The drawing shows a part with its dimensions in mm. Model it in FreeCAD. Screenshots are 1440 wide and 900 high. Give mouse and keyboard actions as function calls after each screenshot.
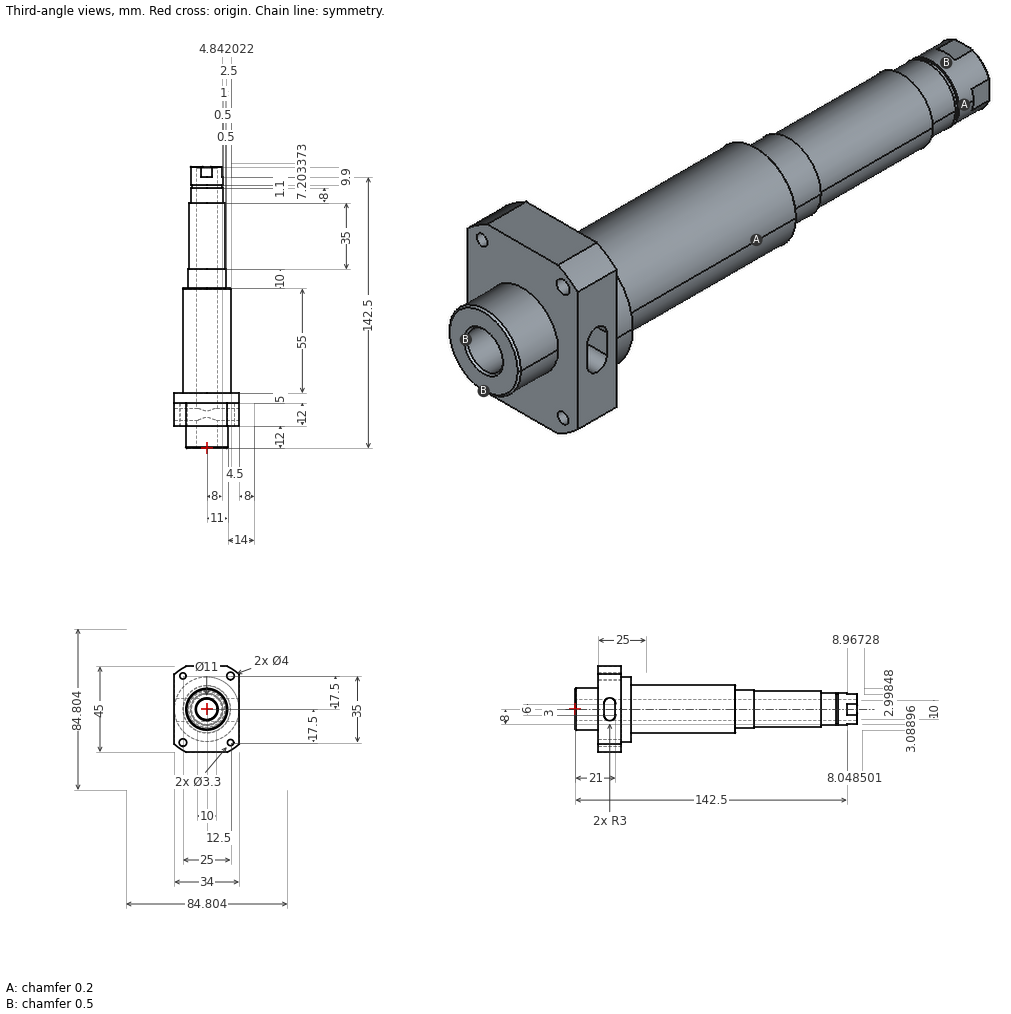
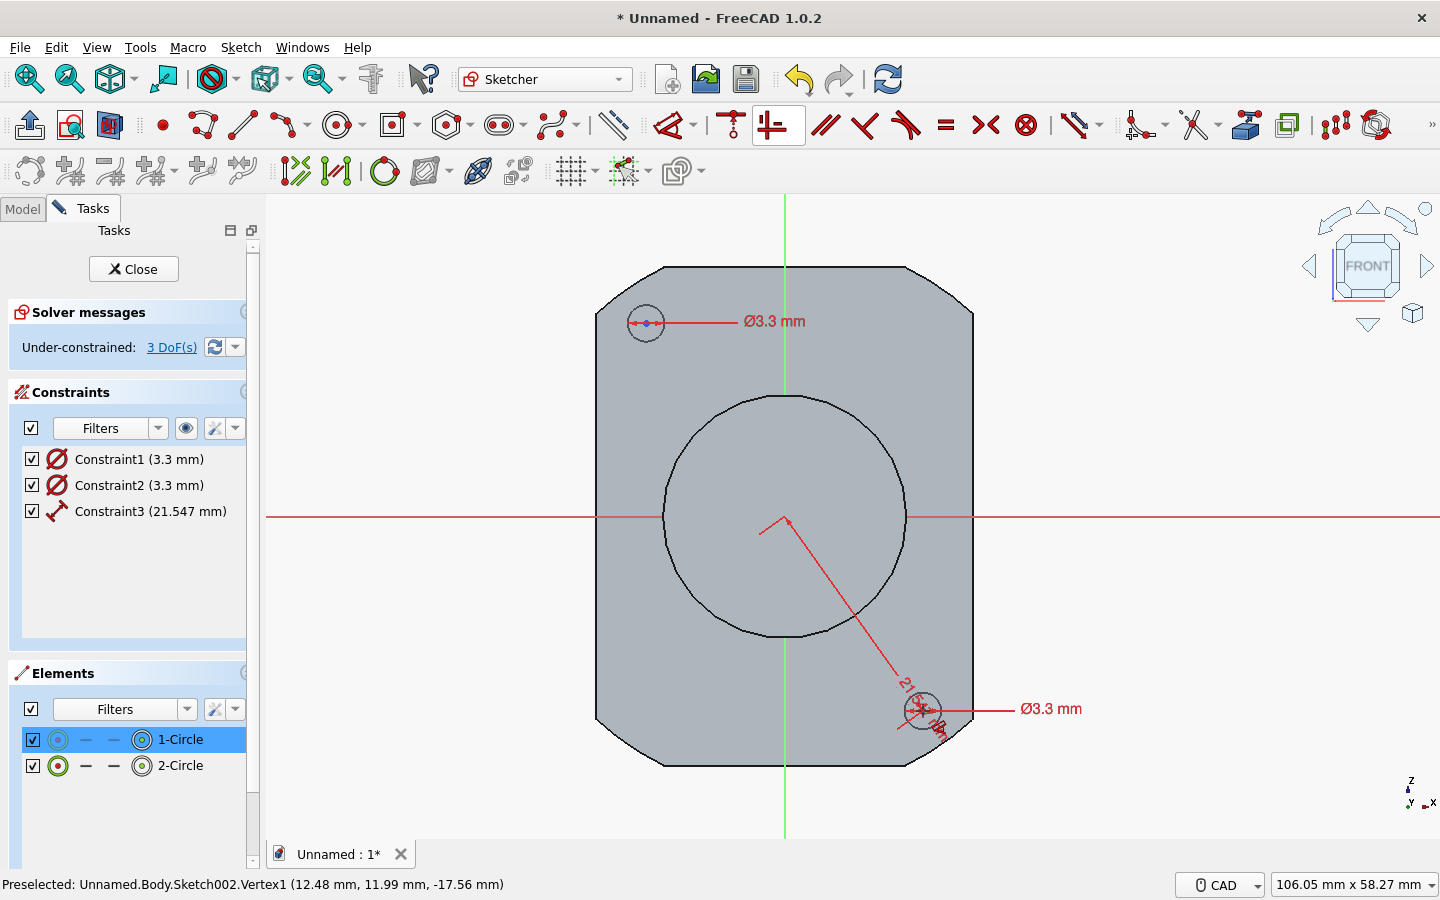
click(646, 323)
click(721, 745)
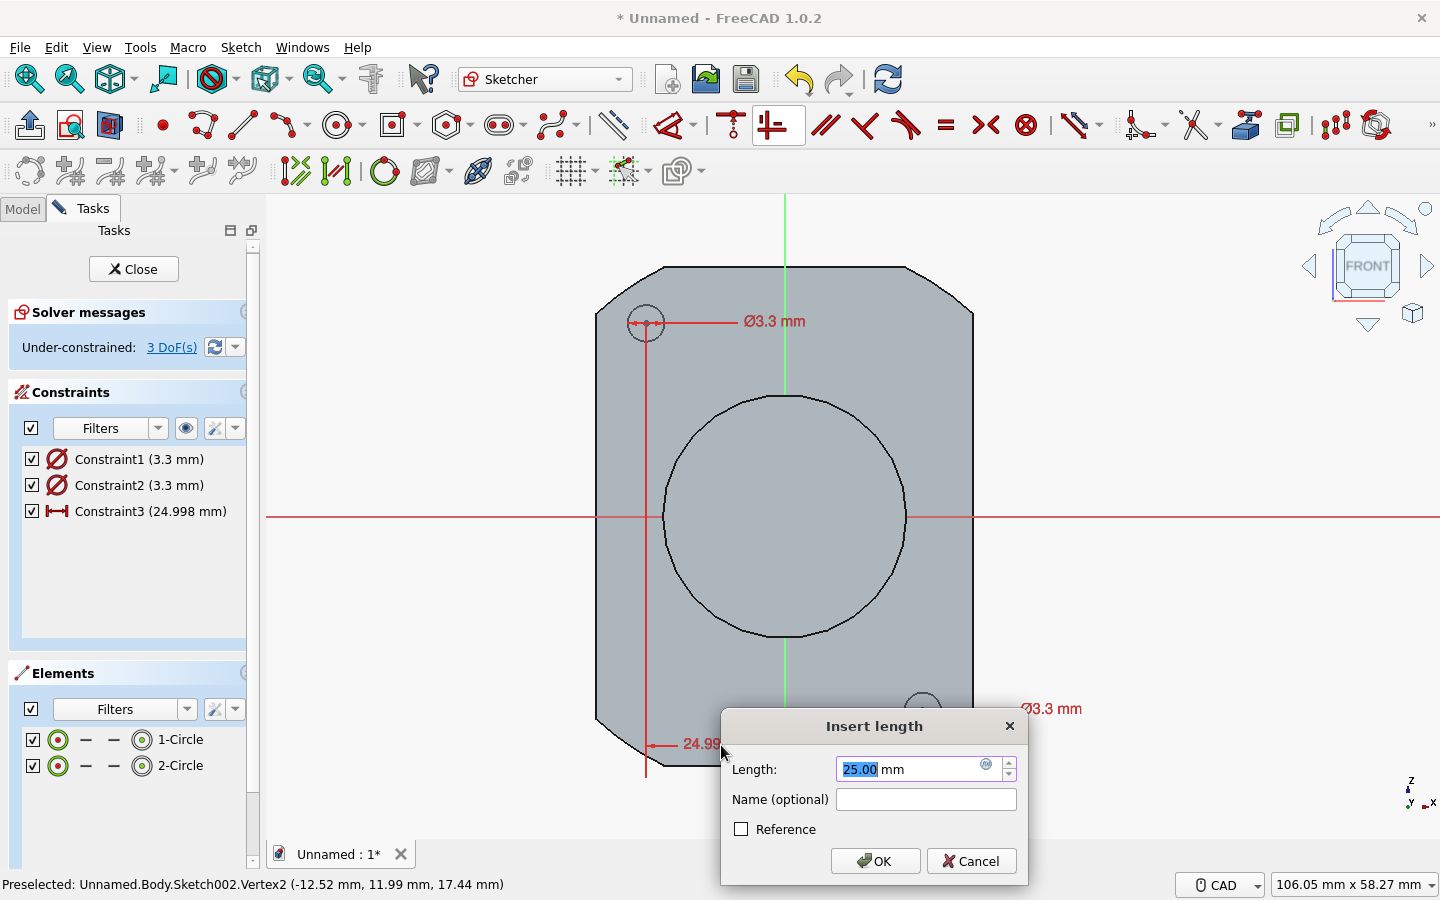
text(25)
key(Return)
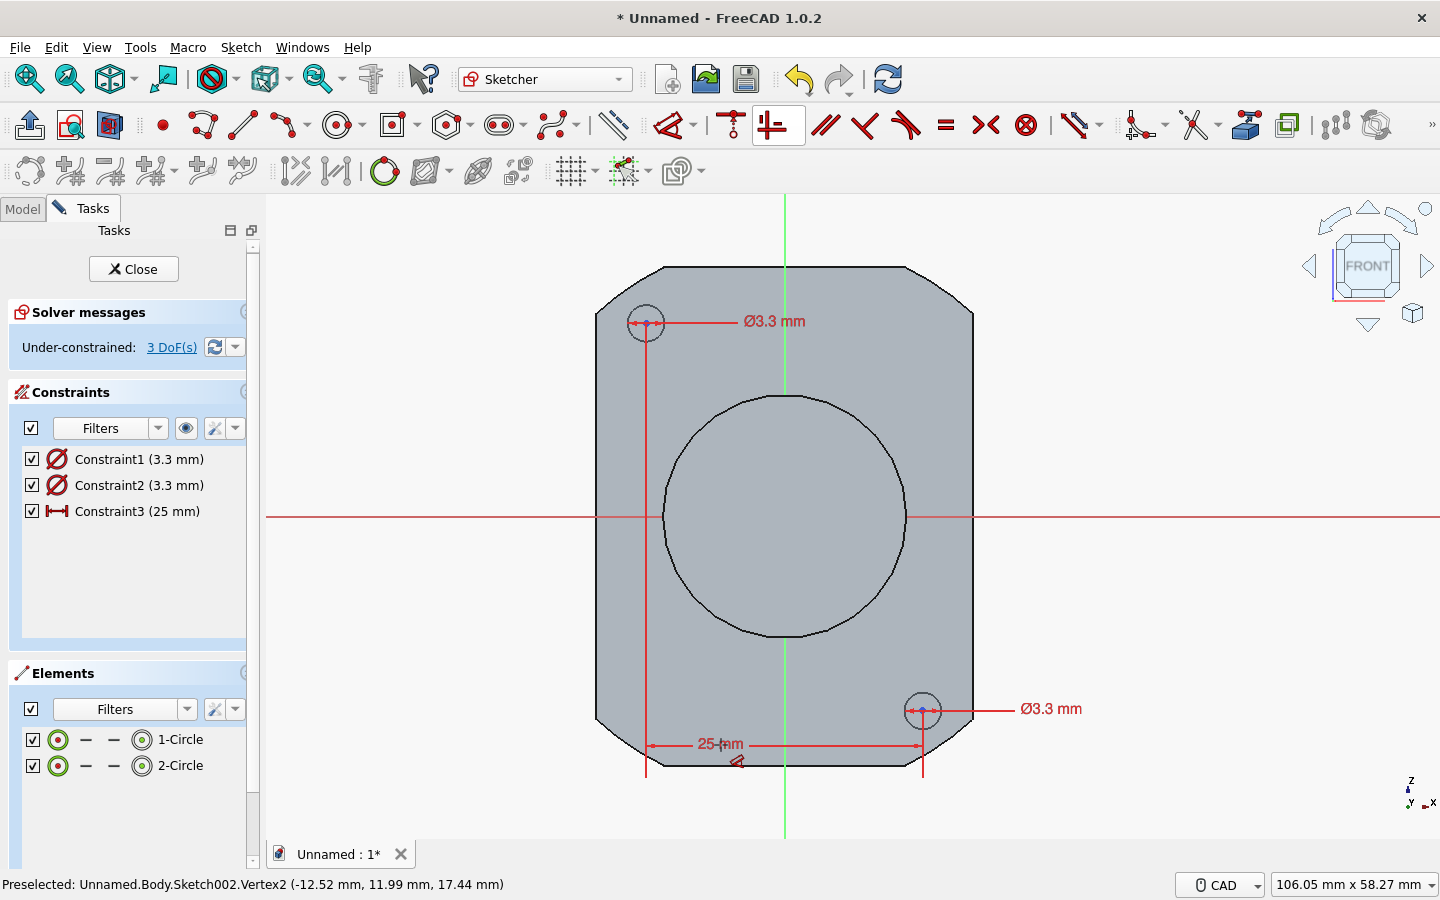
click(923, 711)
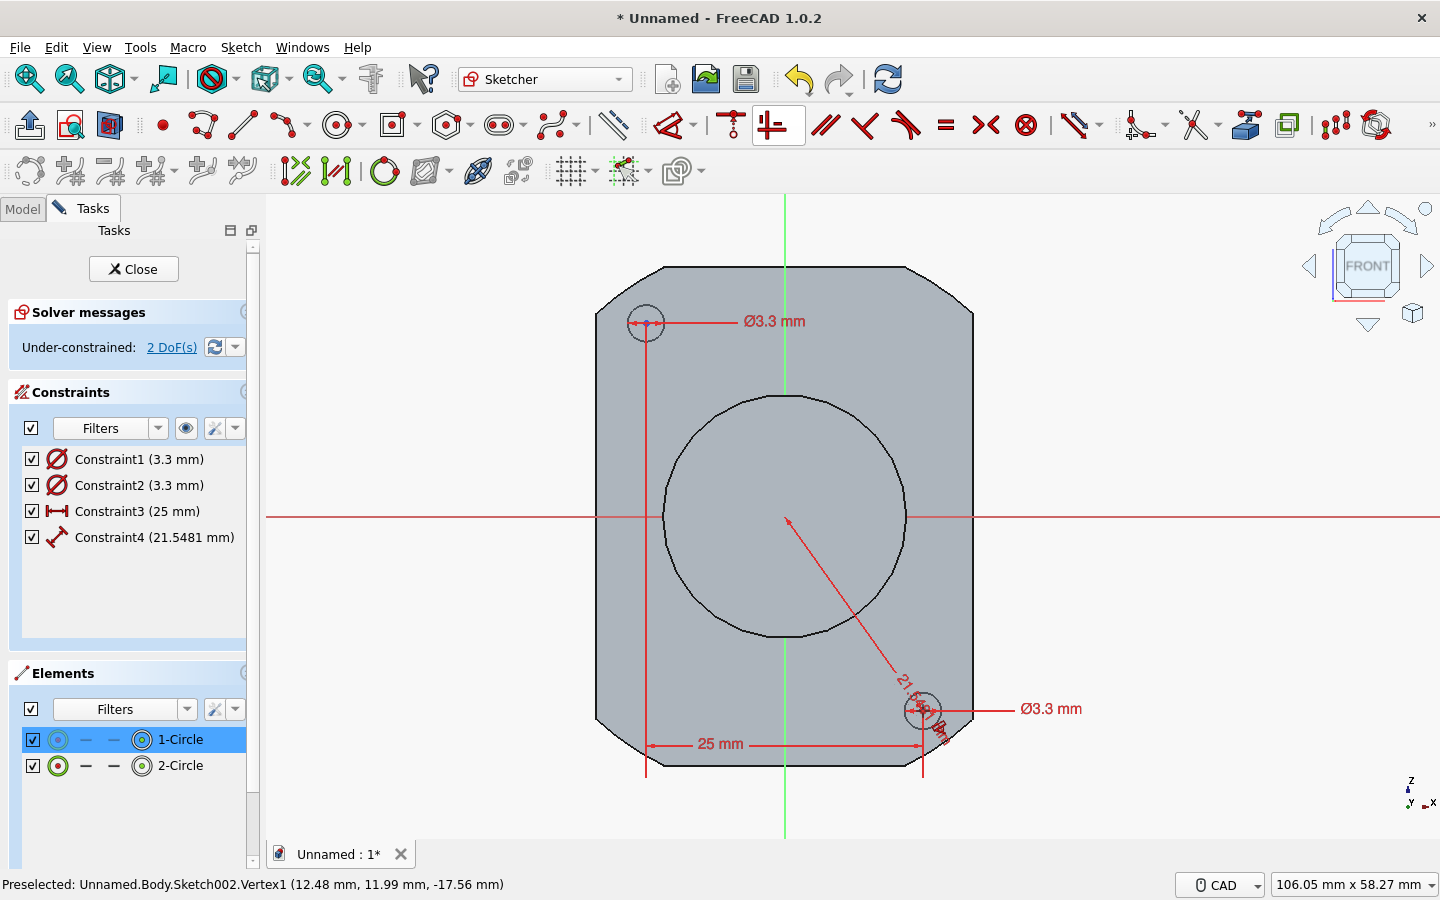
click(646, 323)
click(612, 428)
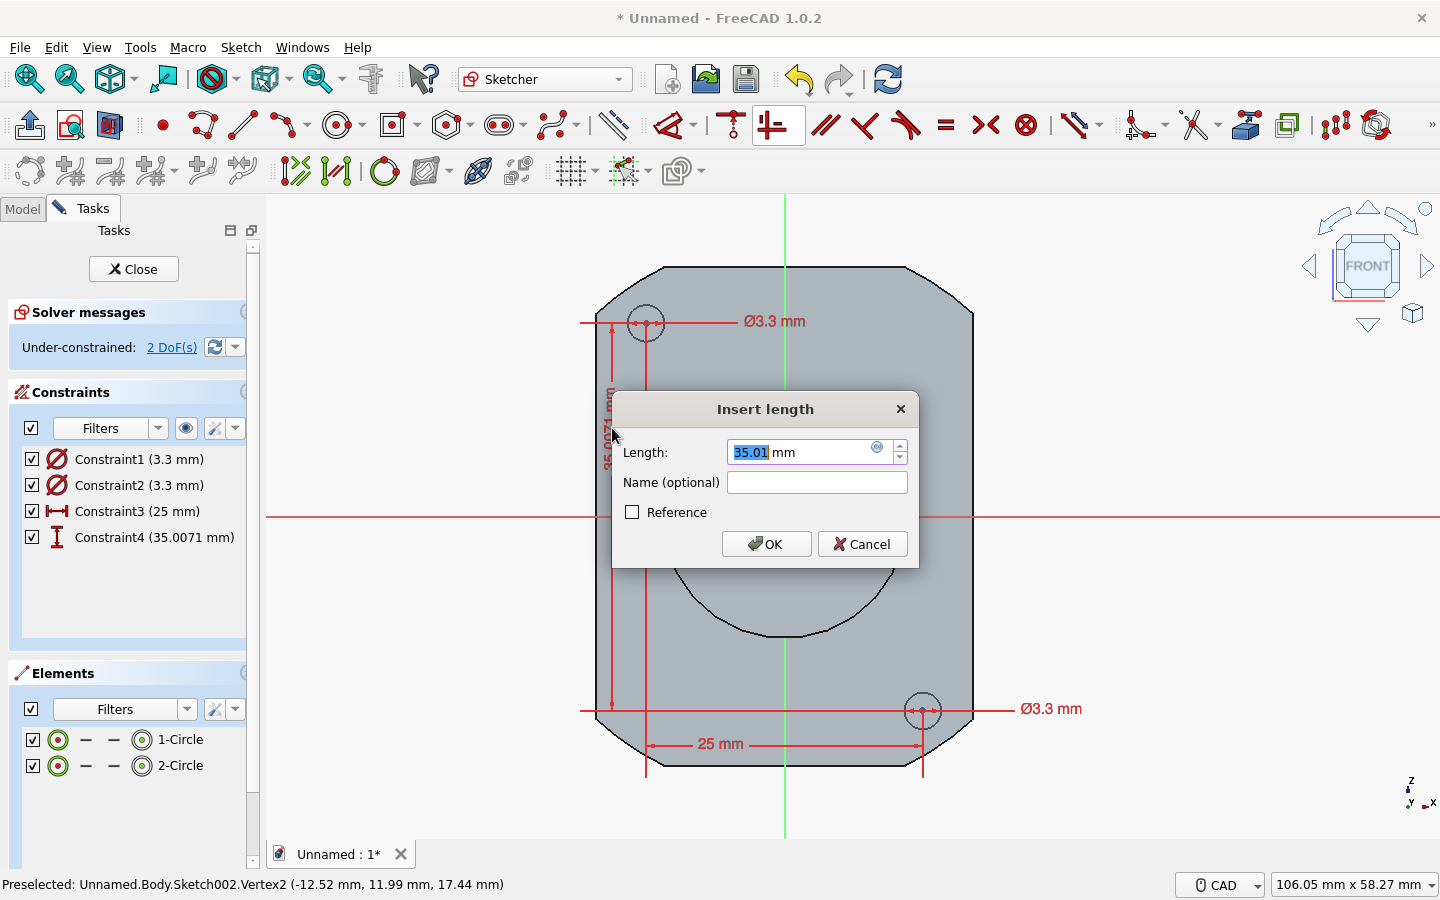
text(35)
key(Return)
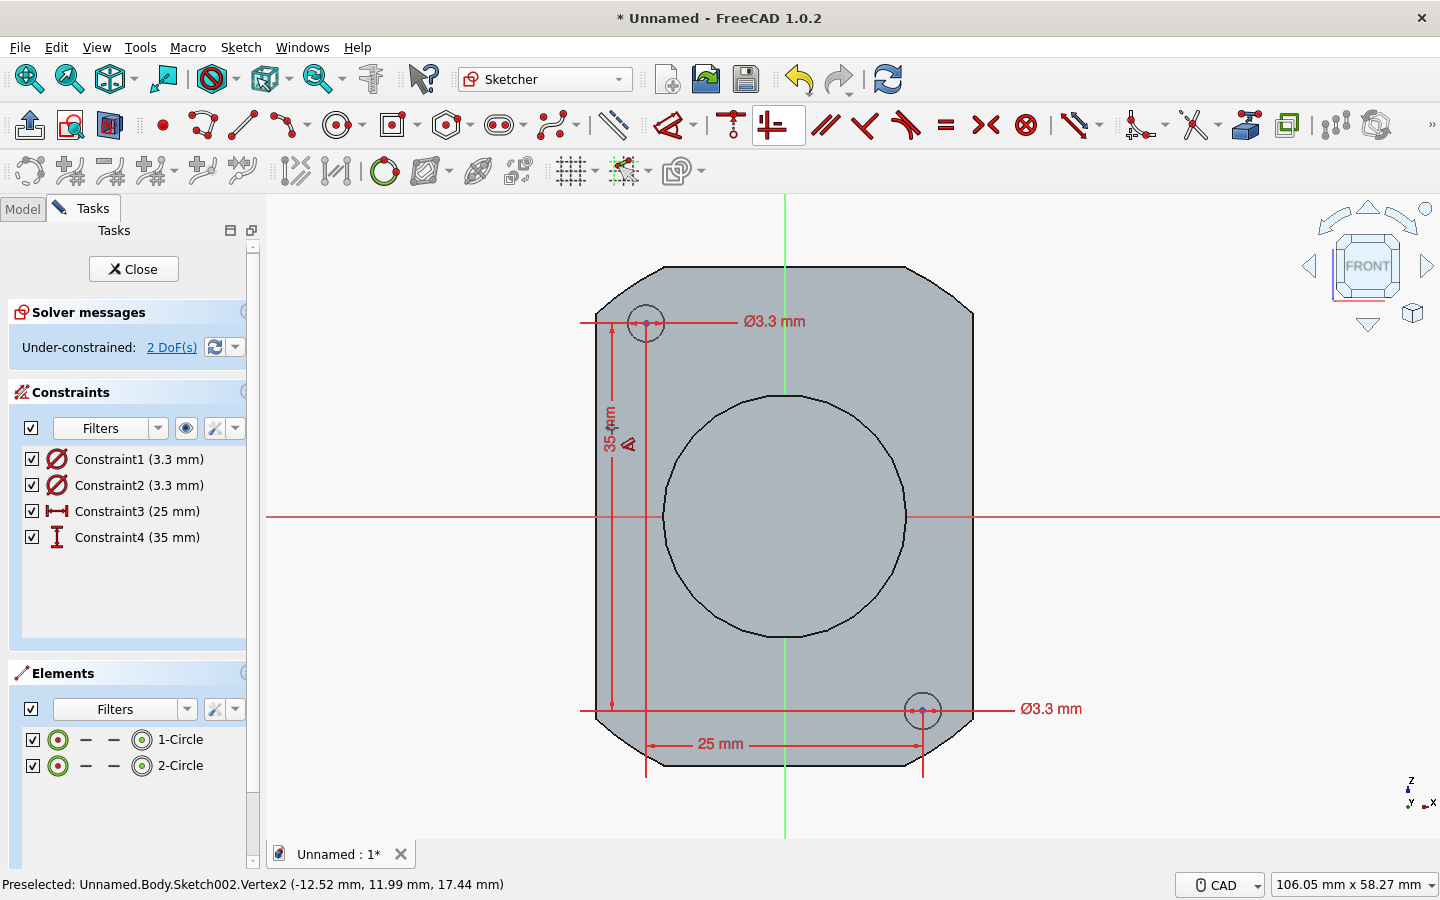
click(923, 711)
click(854, 745)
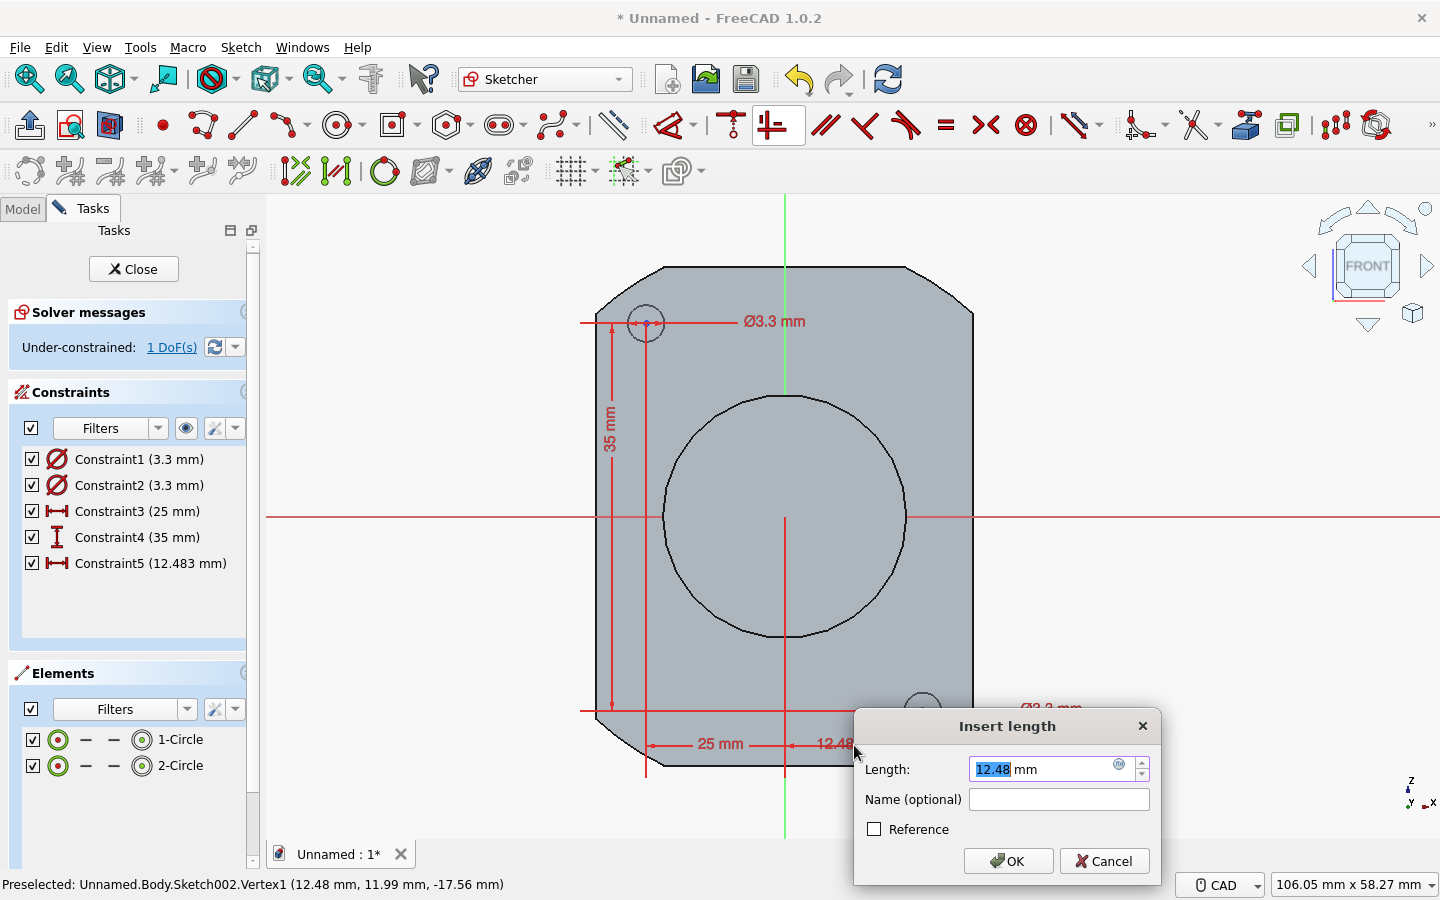
text(12.5)
key(Return)